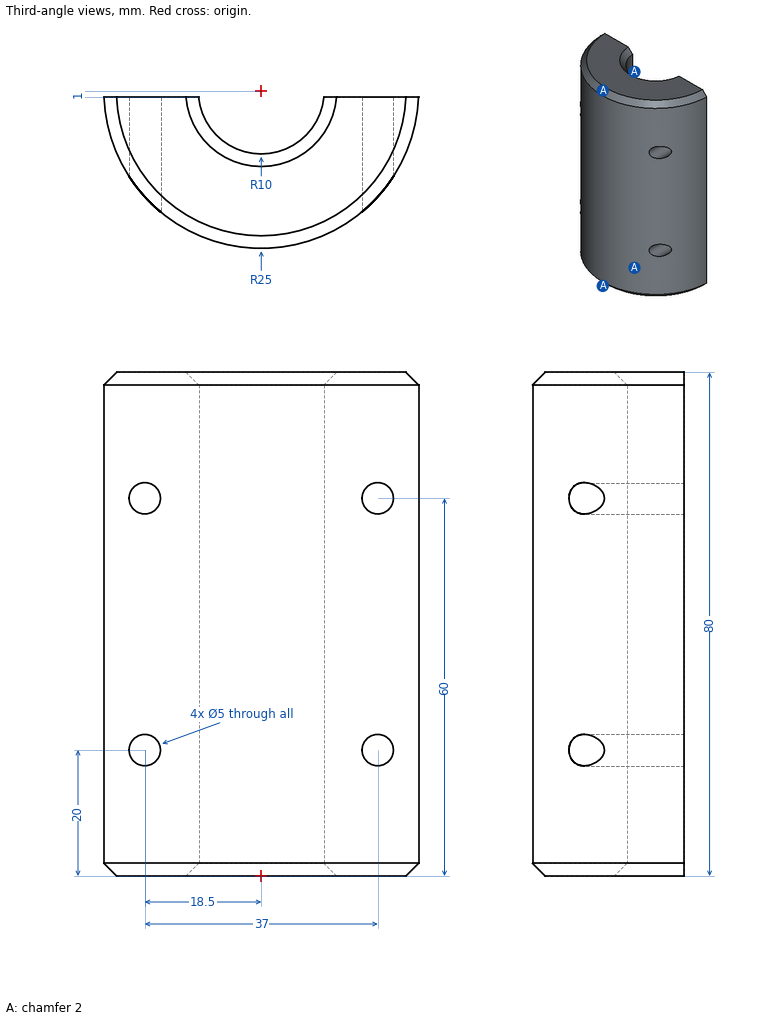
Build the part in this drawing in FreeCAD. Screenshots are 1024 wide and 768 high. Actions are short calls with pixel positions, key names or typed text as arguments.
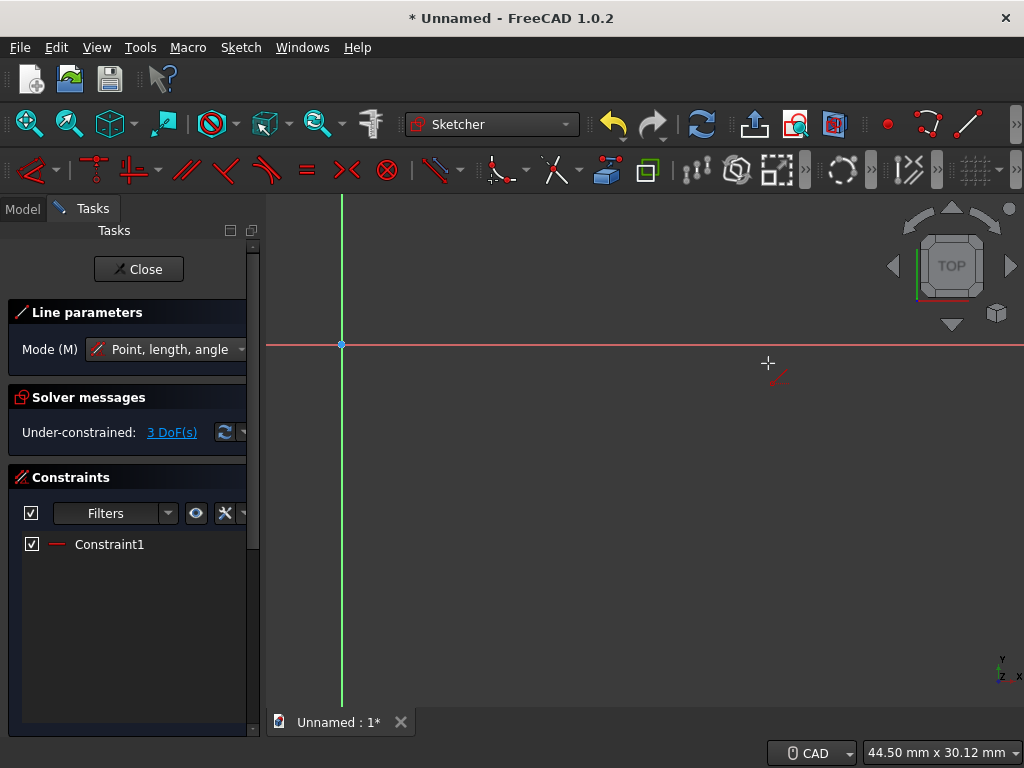
click(767, 362)
click(511, 362)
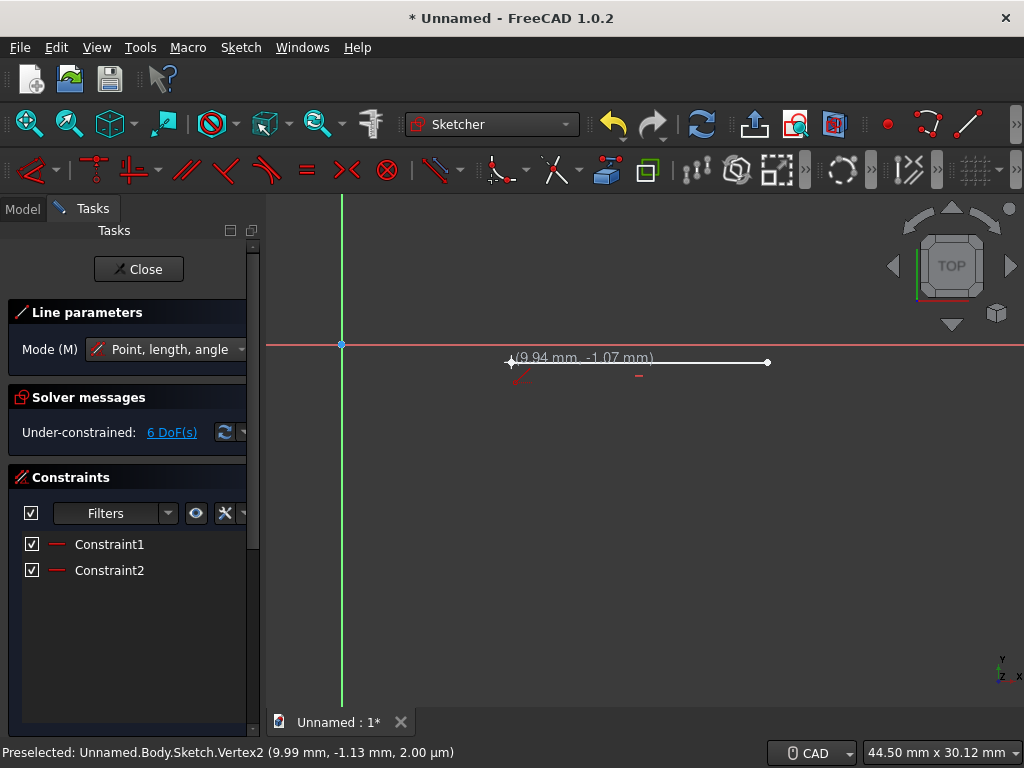
key(g)
key(3)
key(a)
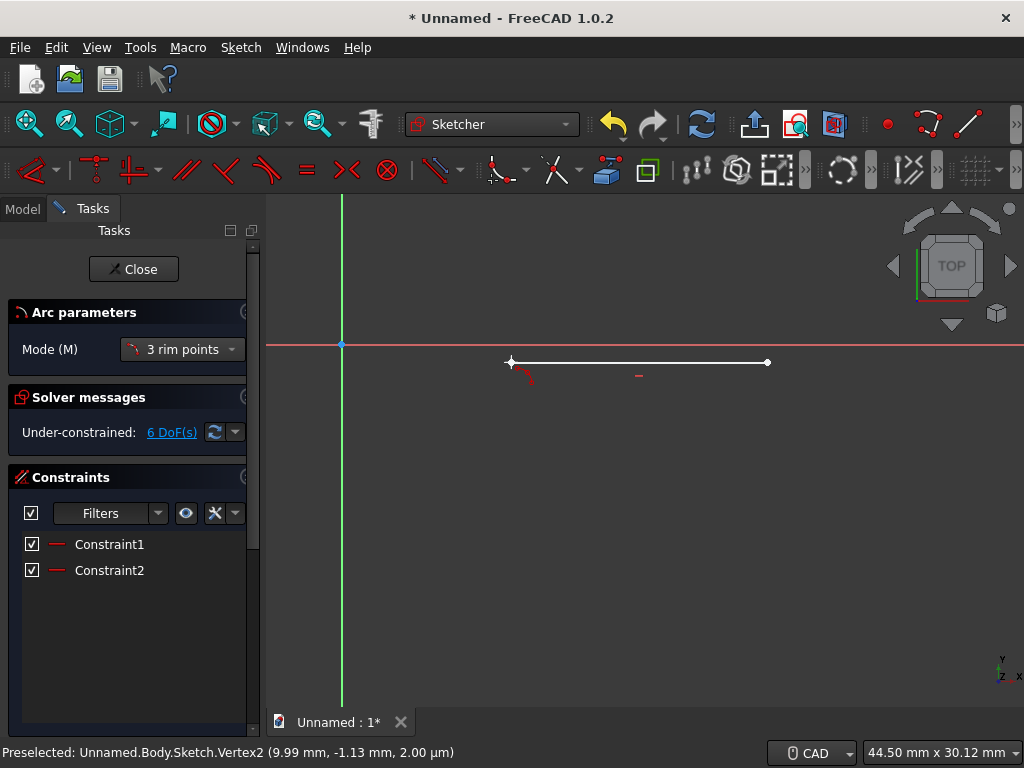
scroll(768, 363, down, 4)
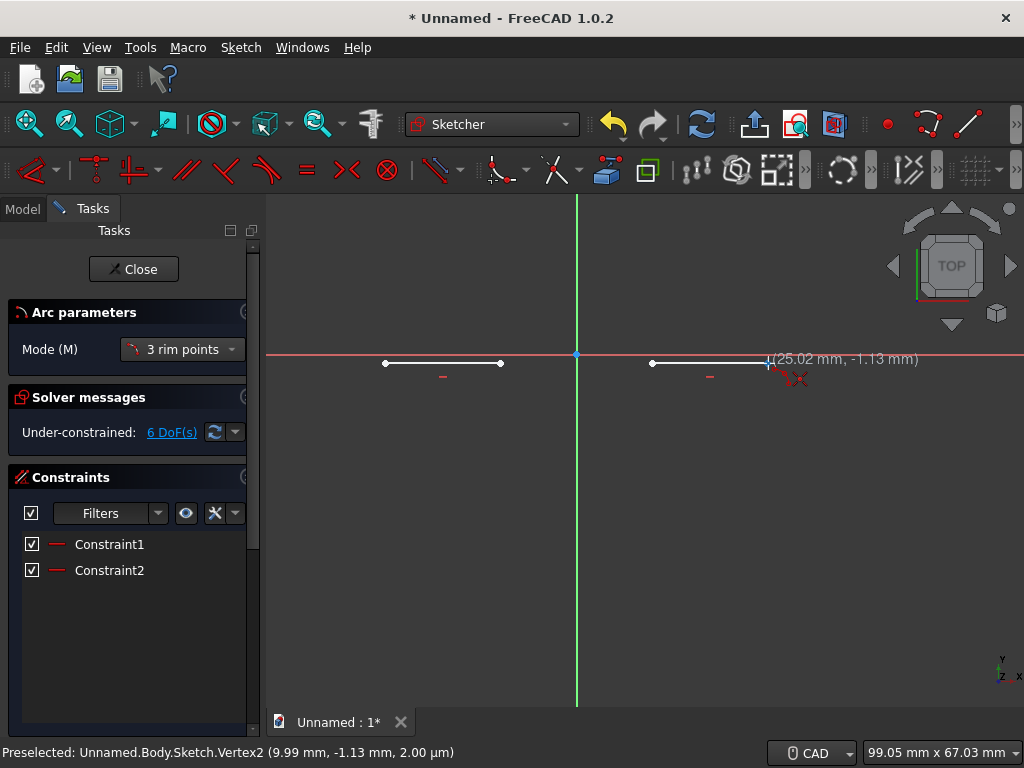
scroll(386, 363, up, 4)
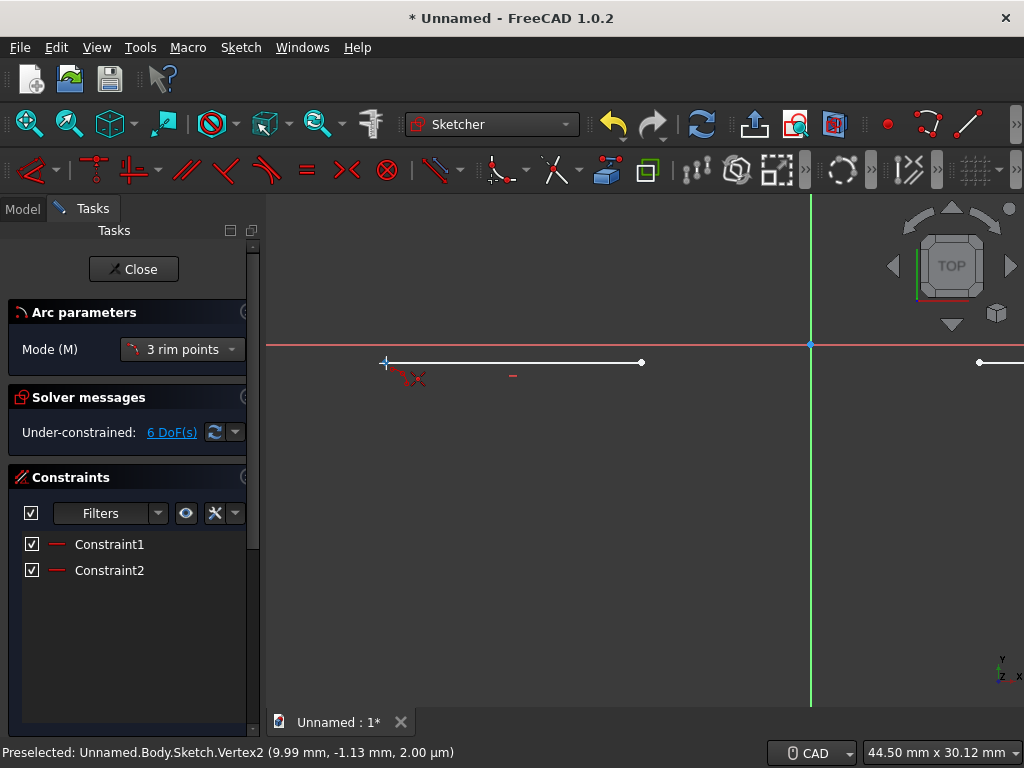
click(385, 363)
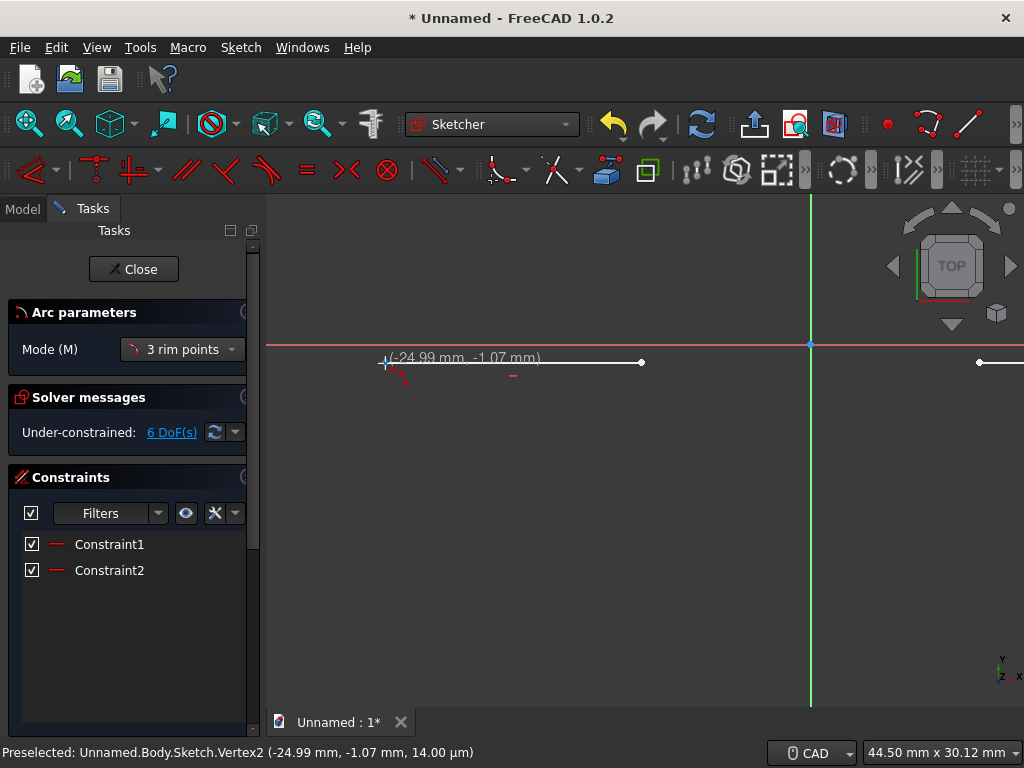
scroll(386, 363, down, 4)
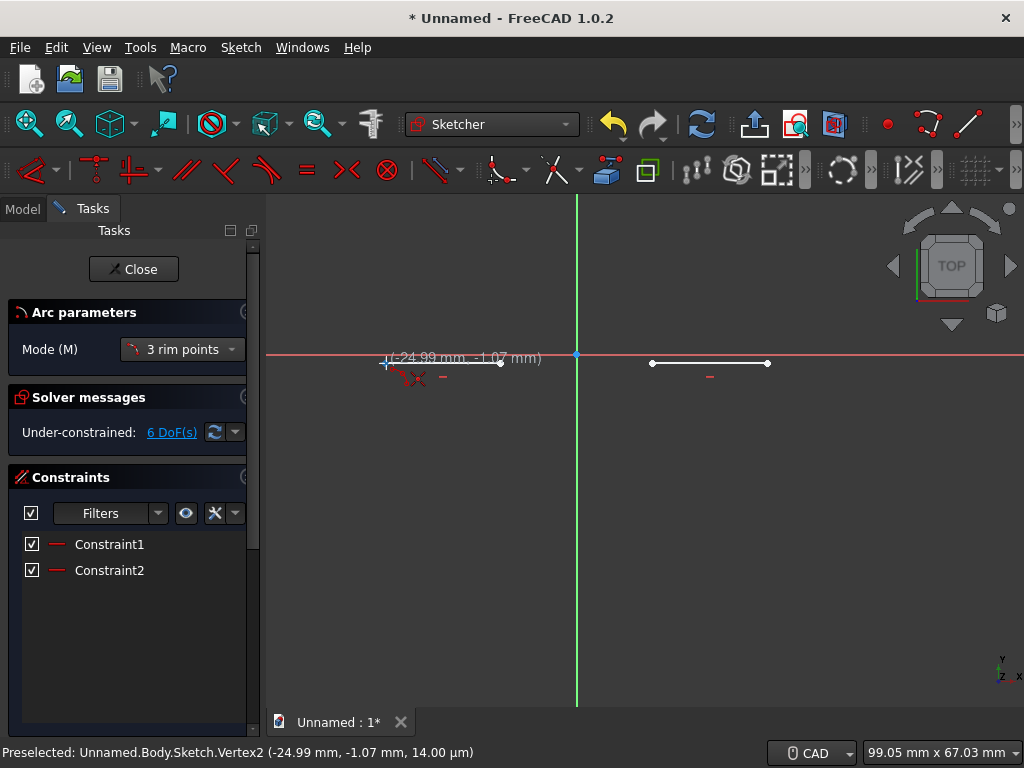
scroll(768, 363, up, 4)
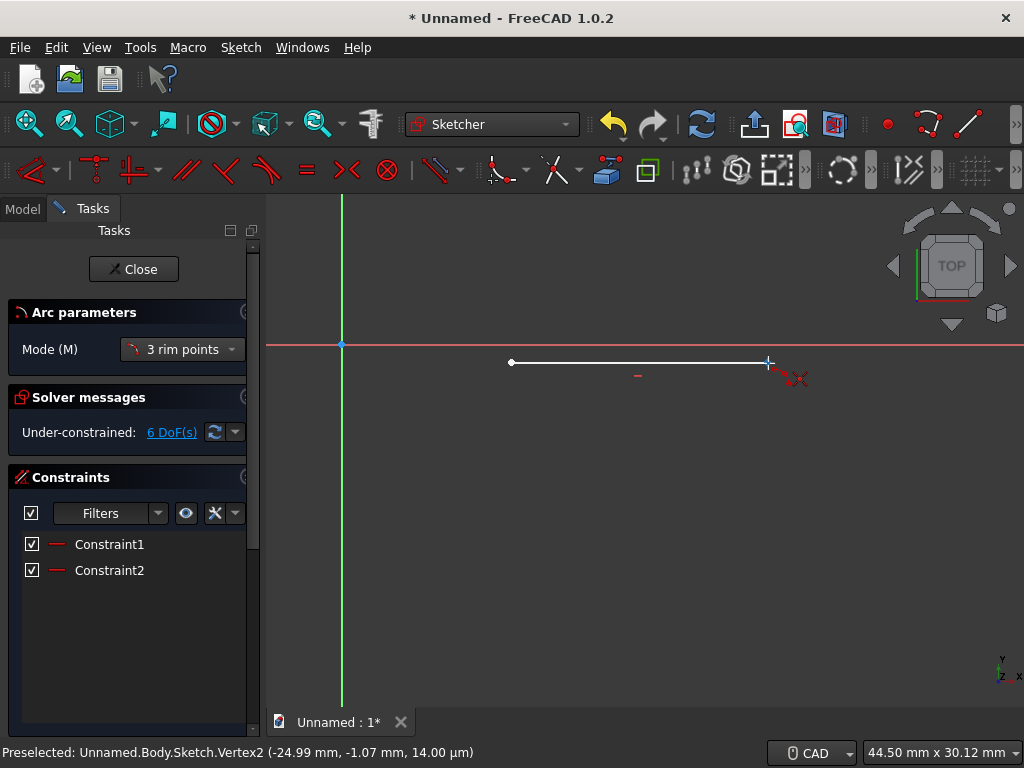
click(767, 363)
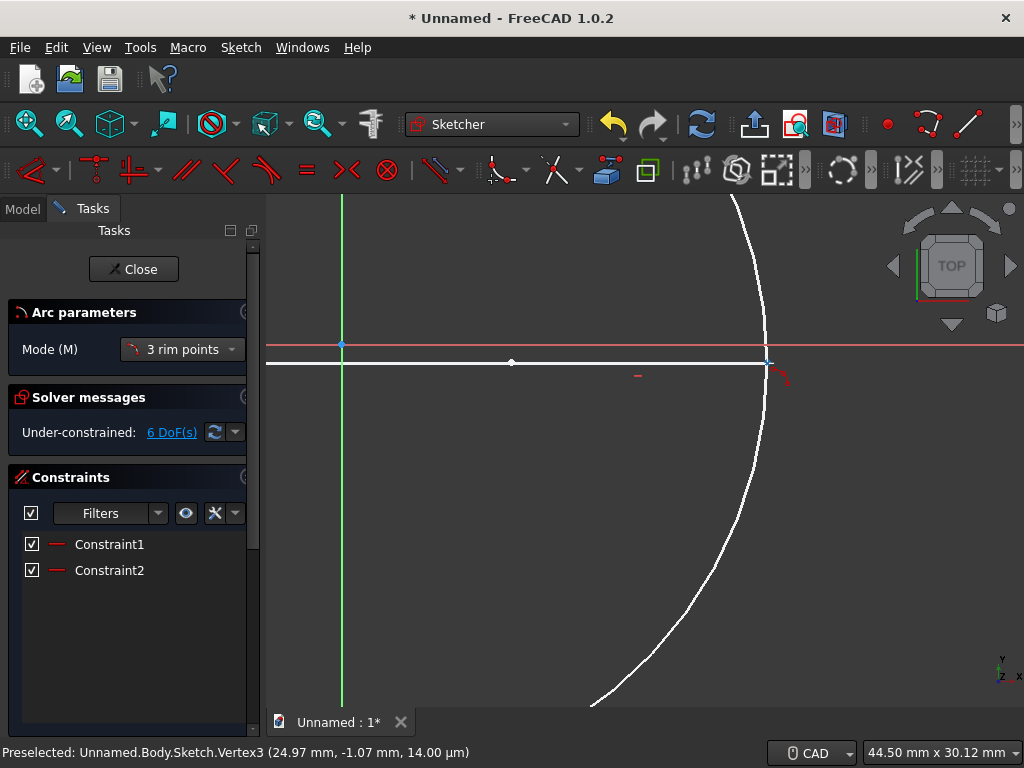
scroll(768, 363, down, 4)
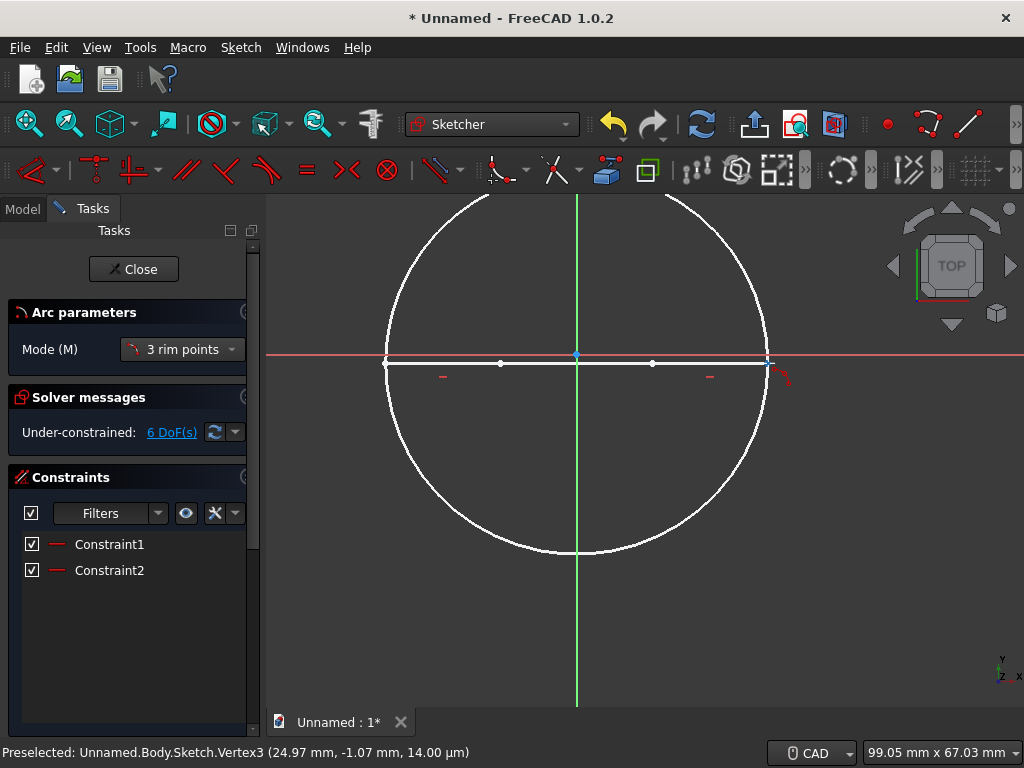
click(519, 537)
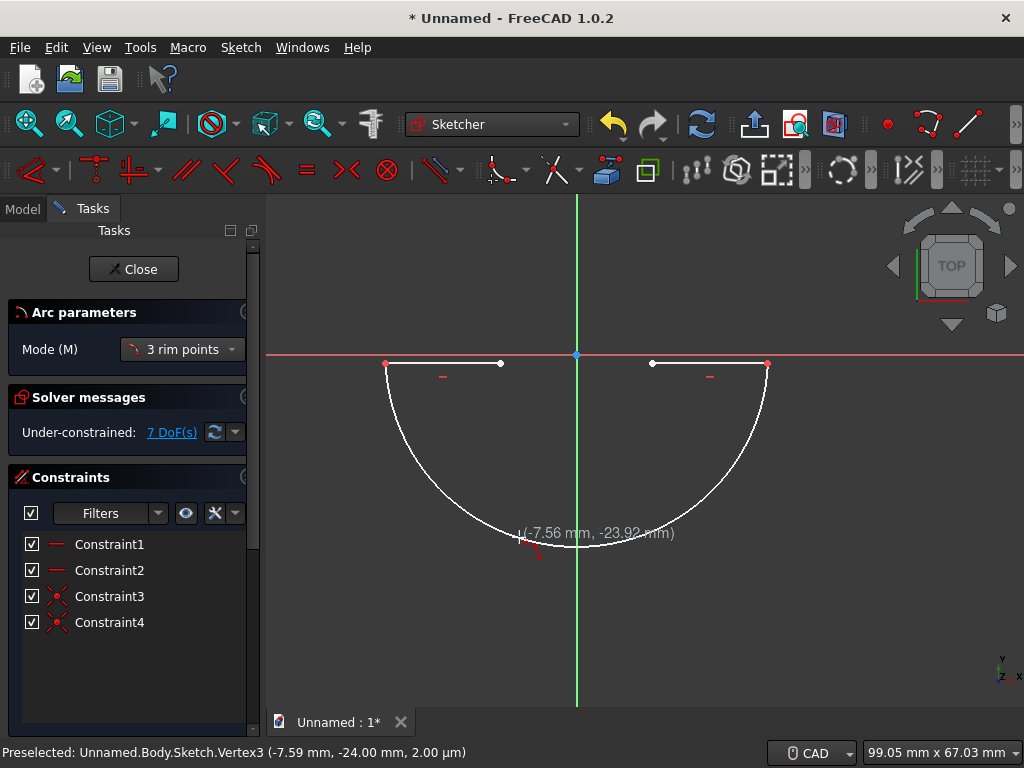
scroll(653, 363, up, 4)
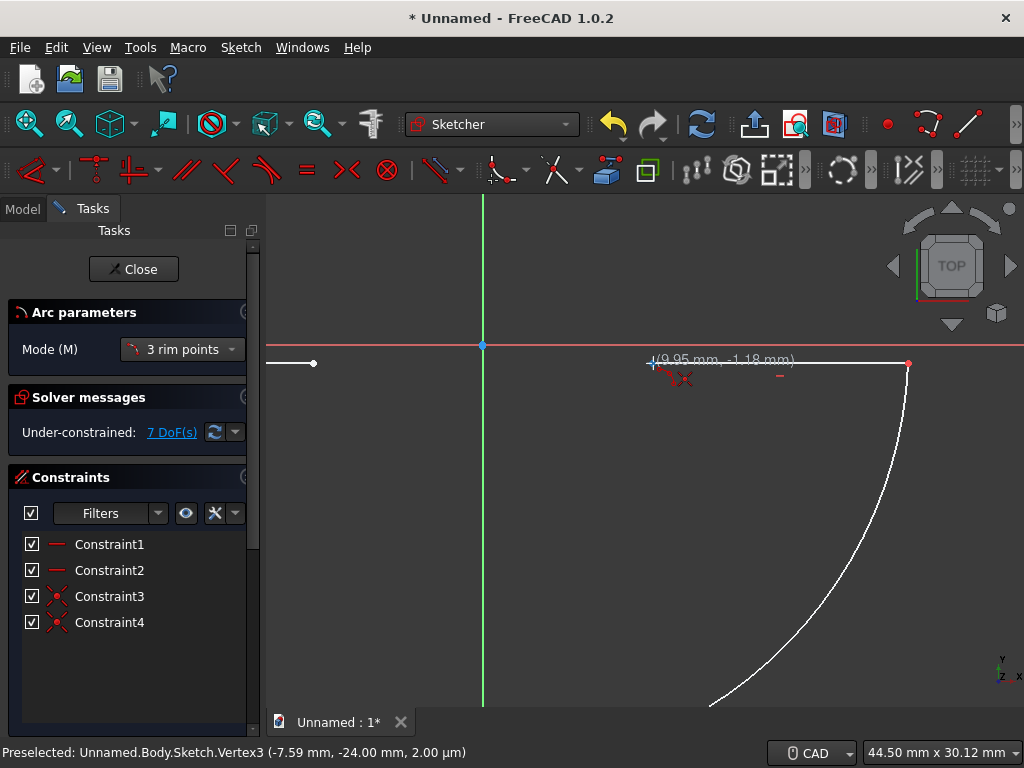
click(652, 363)
click(313, 363)
click(434, 508)
key(Escape)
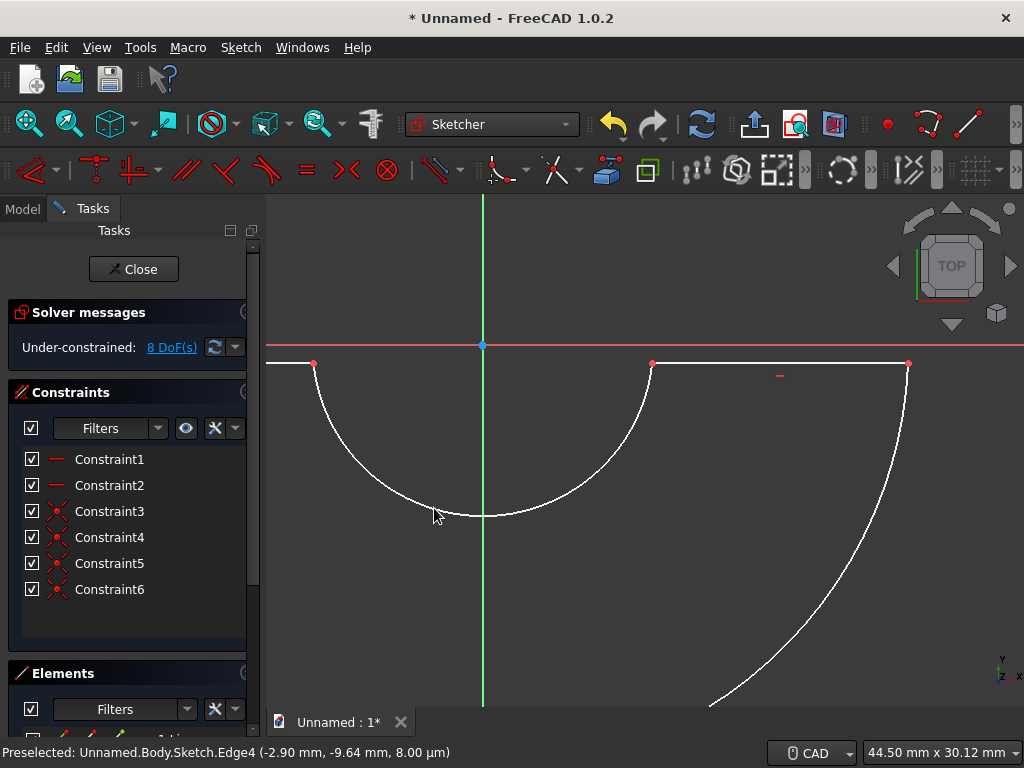
click(821, 605)